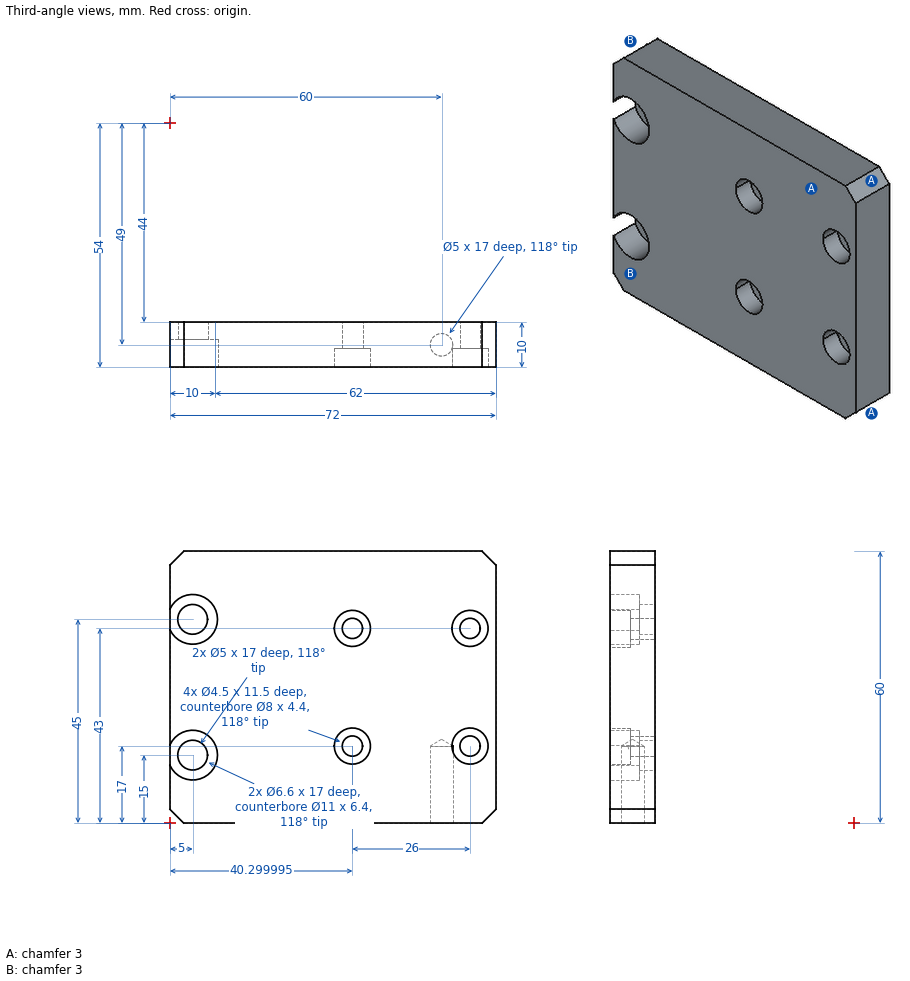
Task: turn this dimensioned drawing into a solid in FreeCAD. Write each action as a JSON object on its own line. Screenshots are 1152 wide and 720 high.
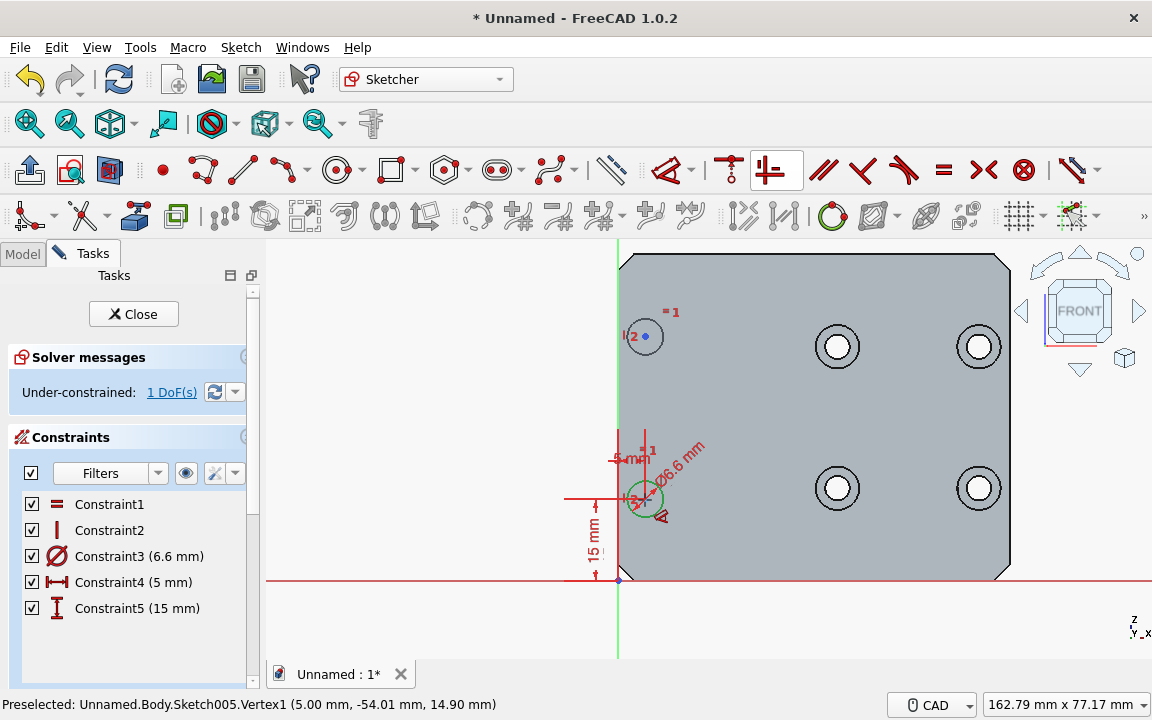
{"action": "left_click", "coordinate": [645, 337]}
{"action": "left_click", "coordinate": [584, 403]}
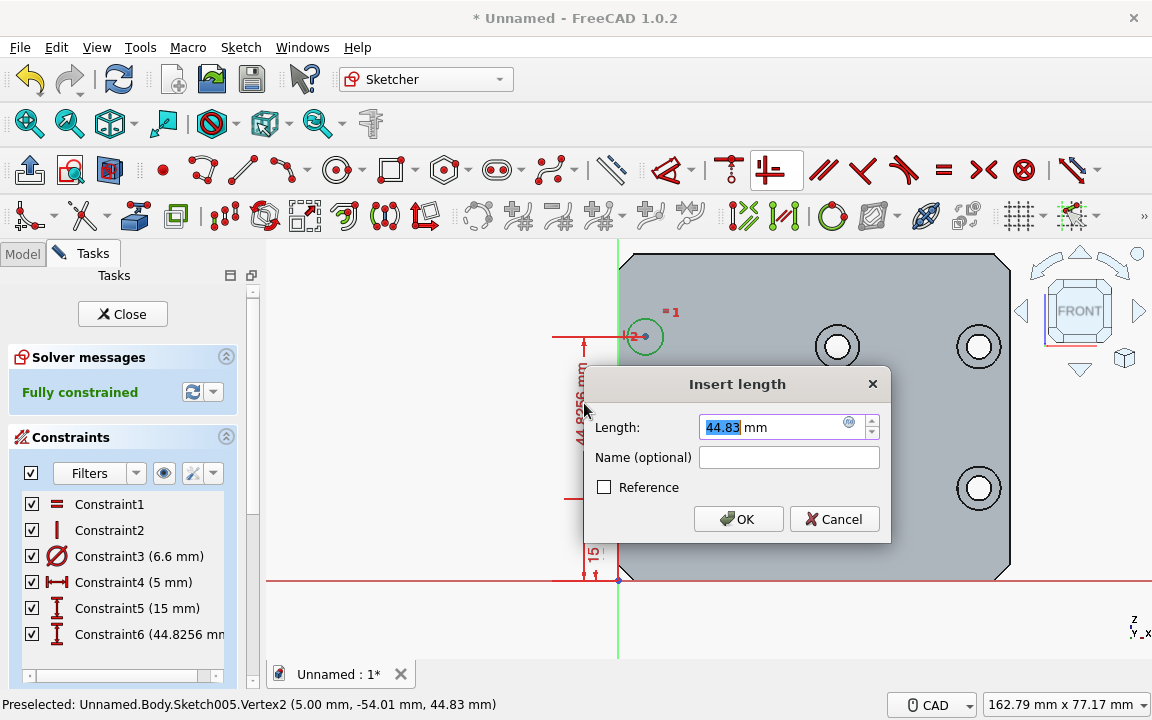
{"action": "type", "text": "45"}
{"action": "key", "text": "Return"}
{"action": "key", "text": "Escape"}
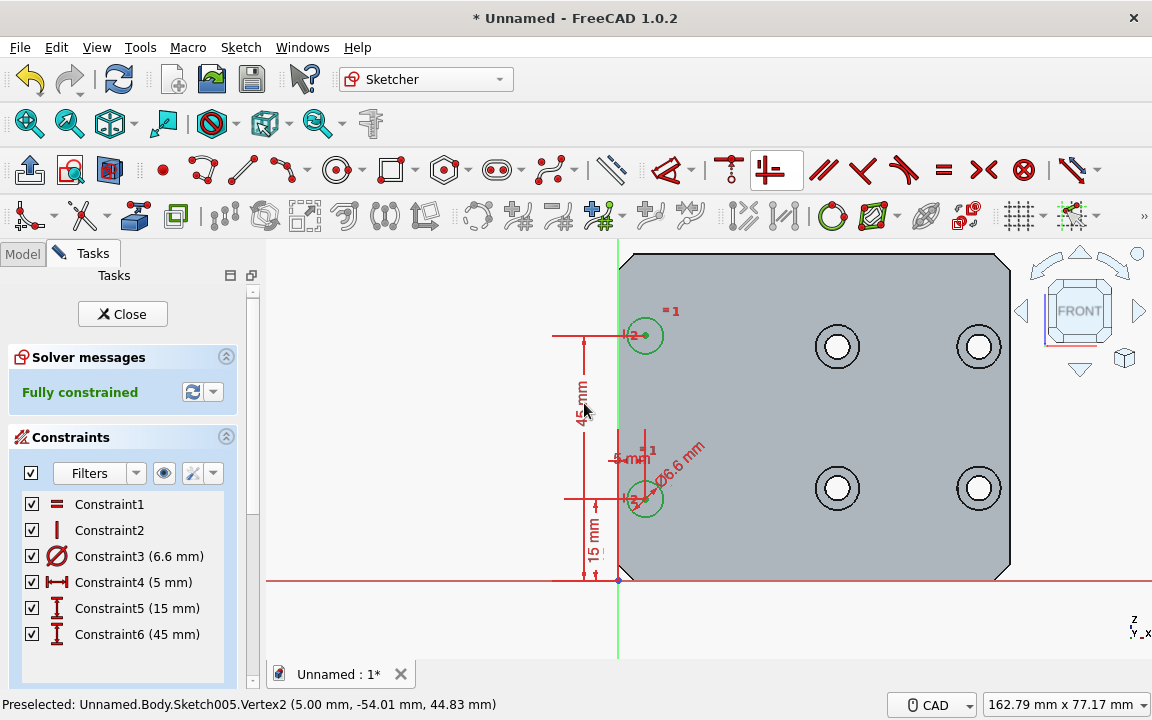
{"action": "left_click", "coordinate": [123, 314]}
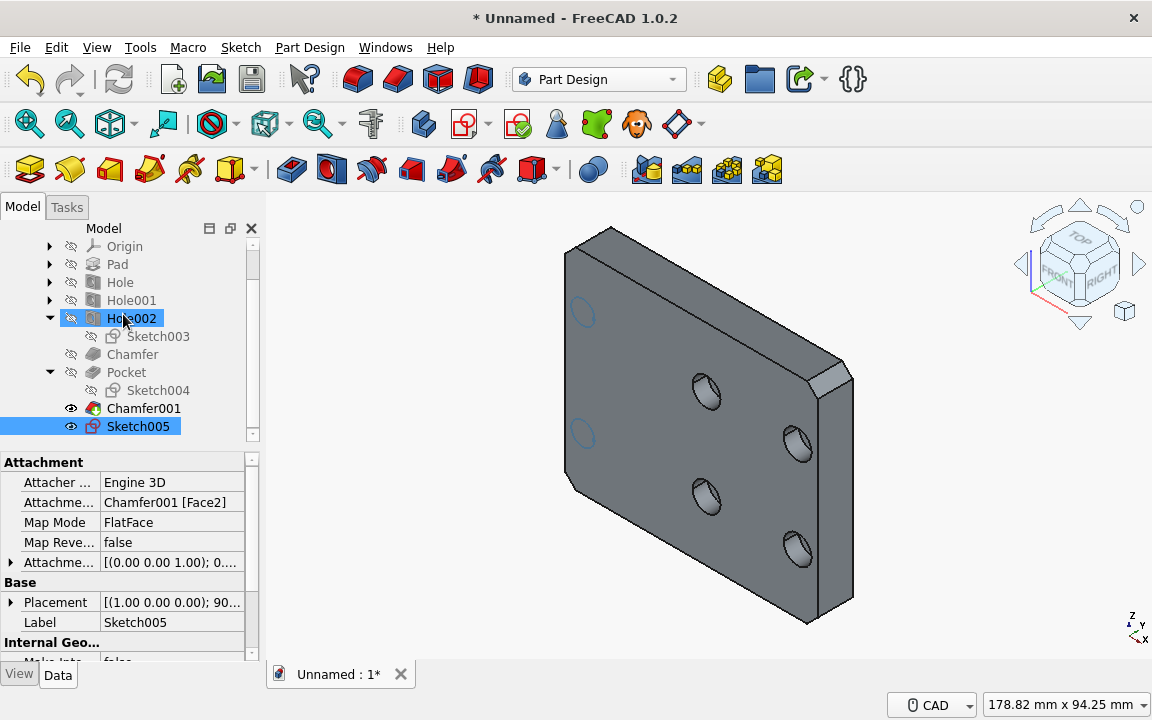
{"action": "left_click", "coordinate": [332, 170]}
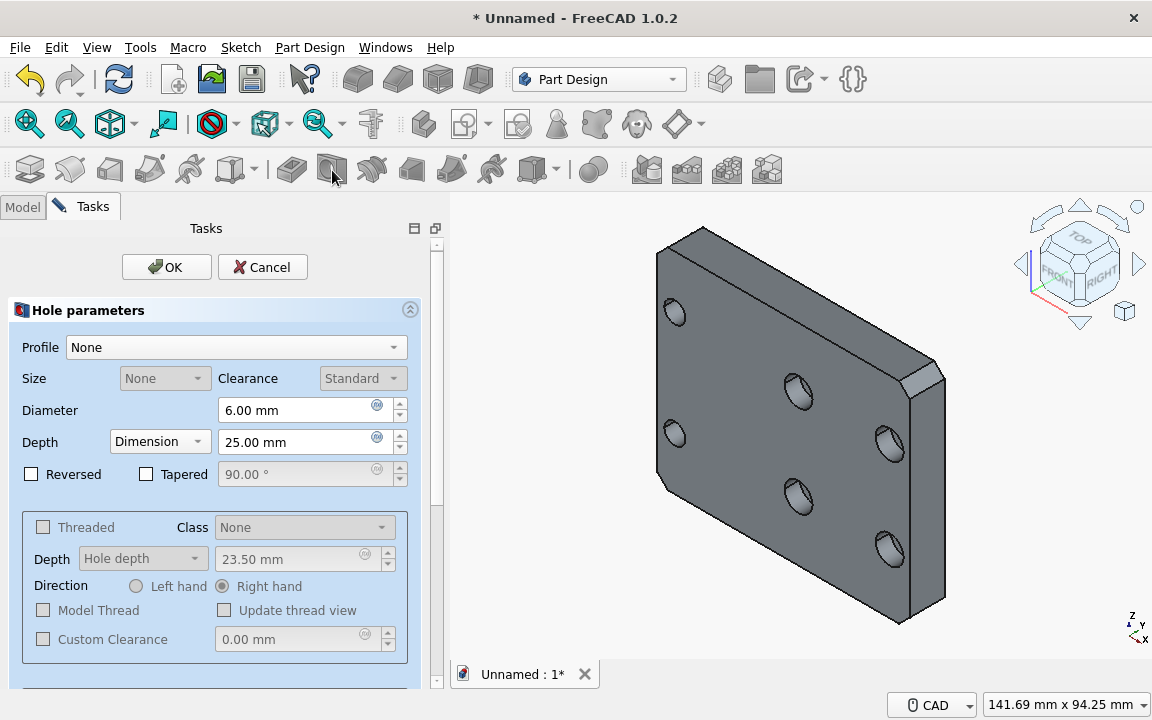
{"action": "triple_click", "coordinate": [305, 410]}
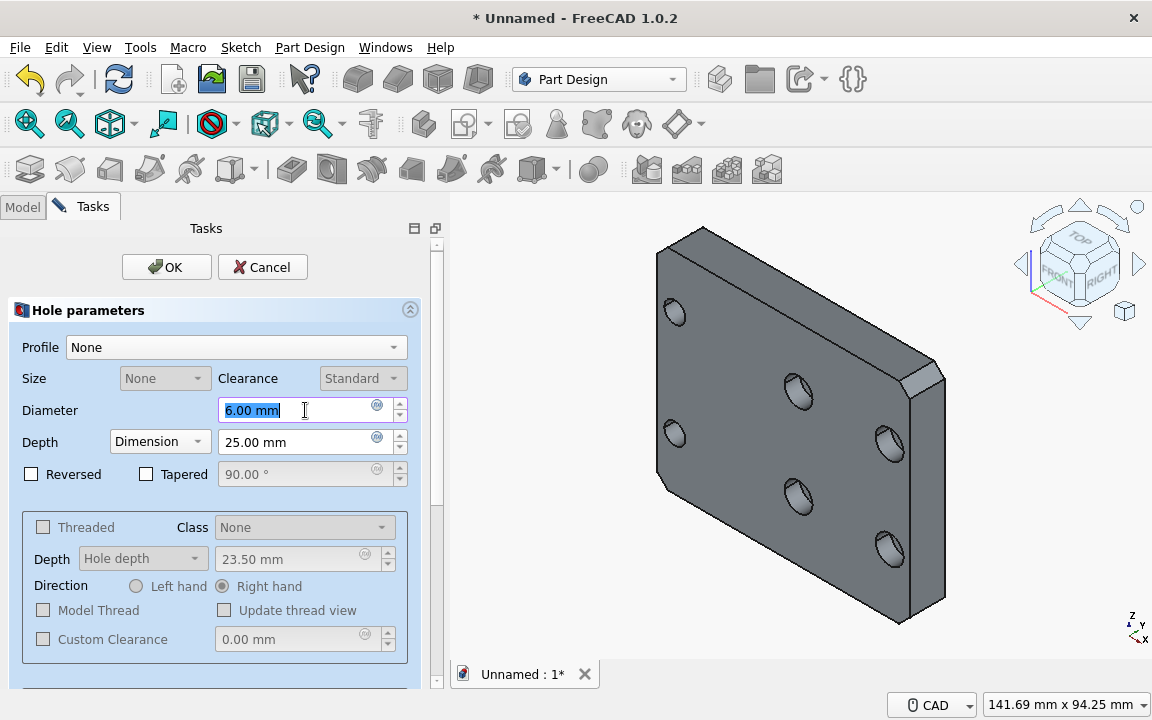
{"action": "type", "text": "6.6"}
{"action": "key", "text": "Tab"}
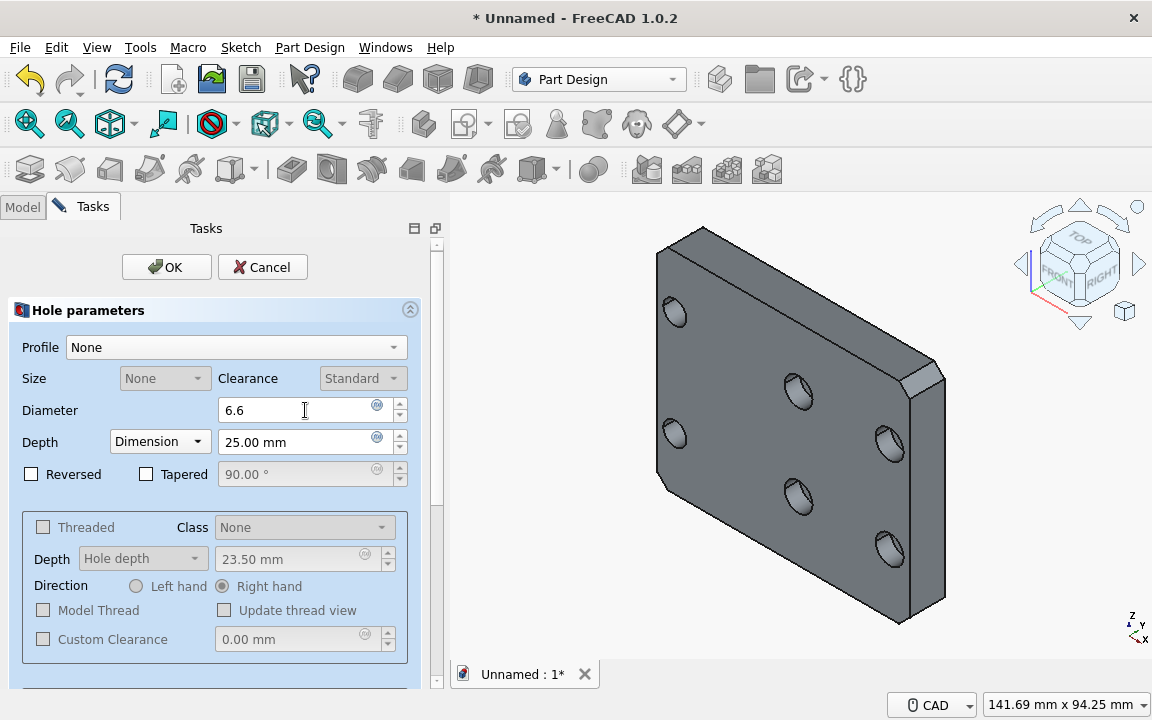
{"action": "triple_click", "coordinate": [305, 442]}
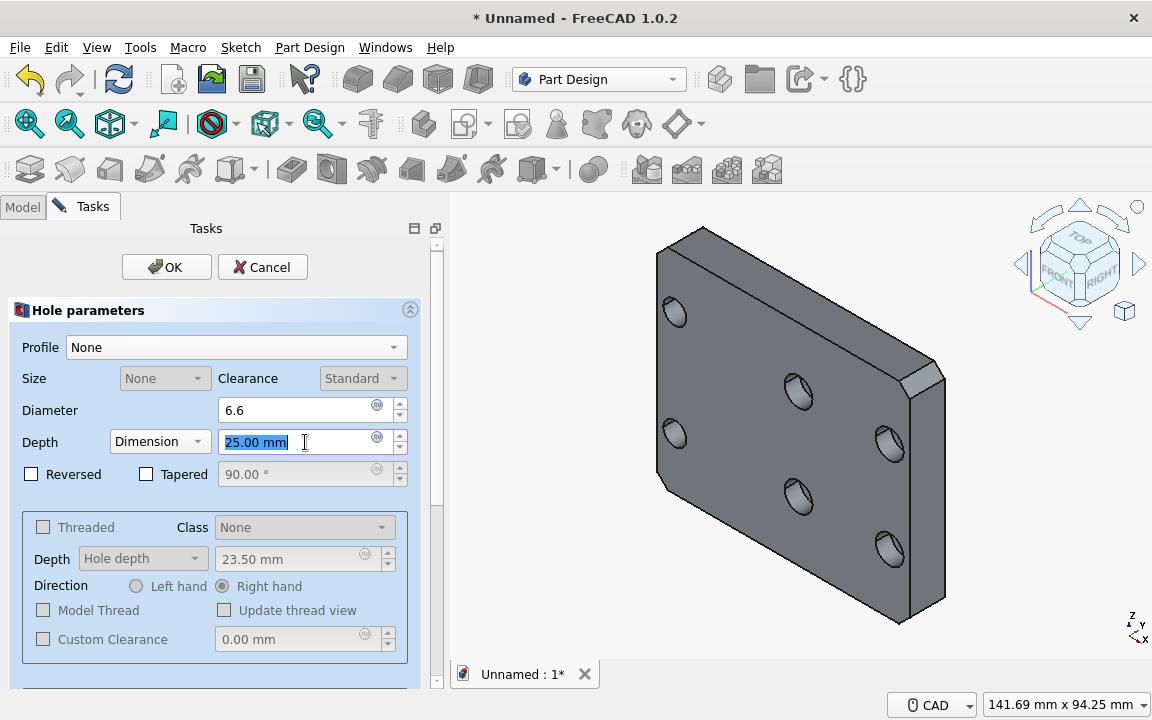
{"action": "type", "text": "17"}
{"action": "key", "text": "Tab"}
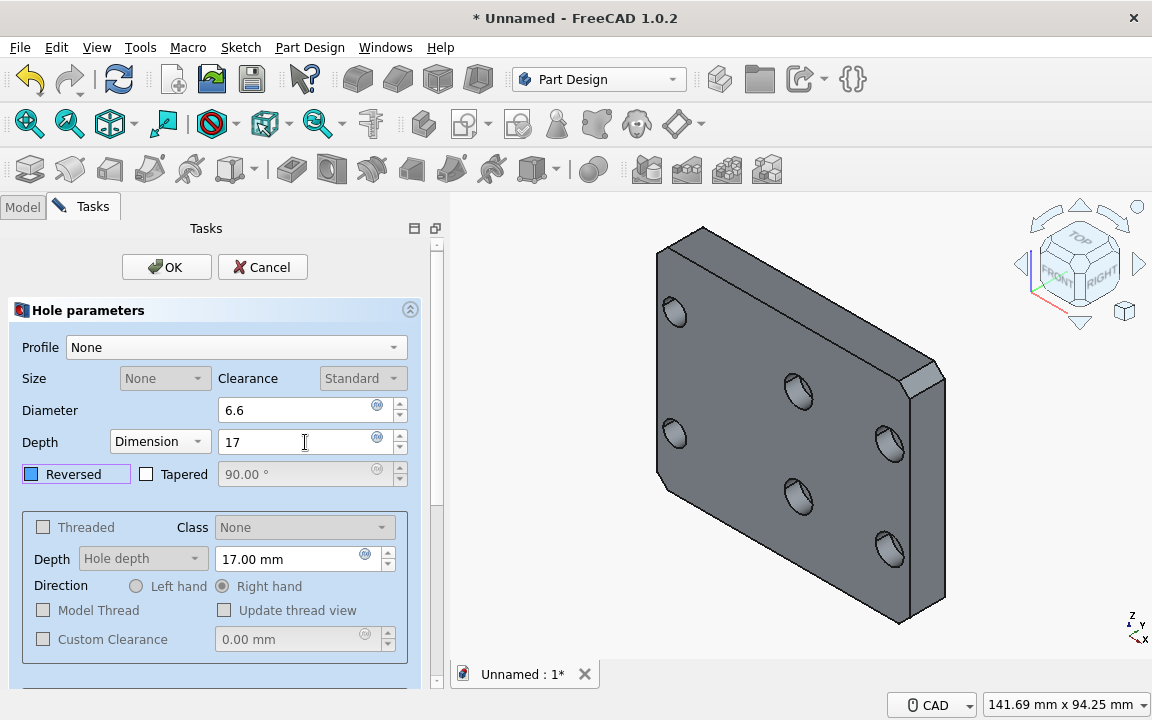
{"action": "scroll", "coordinate": [437, 463], "scroll_direction": "down", "scroll_amount": 2}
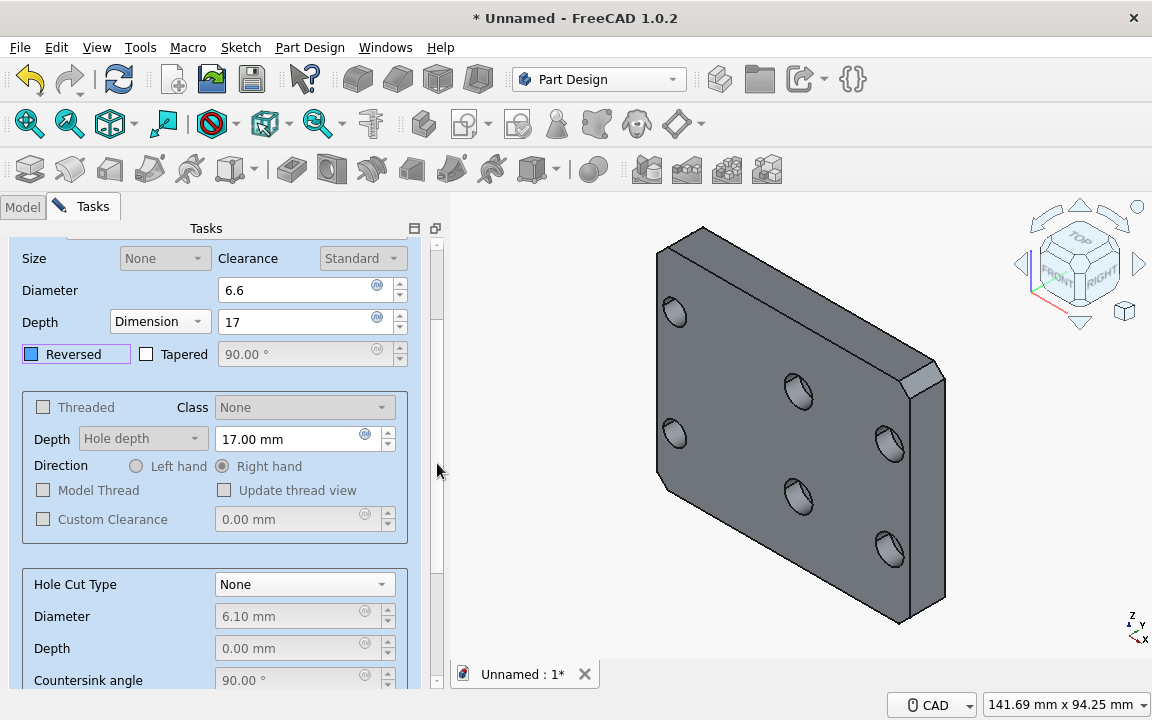
{"action": "left_click", "coordinate": [306, 584]}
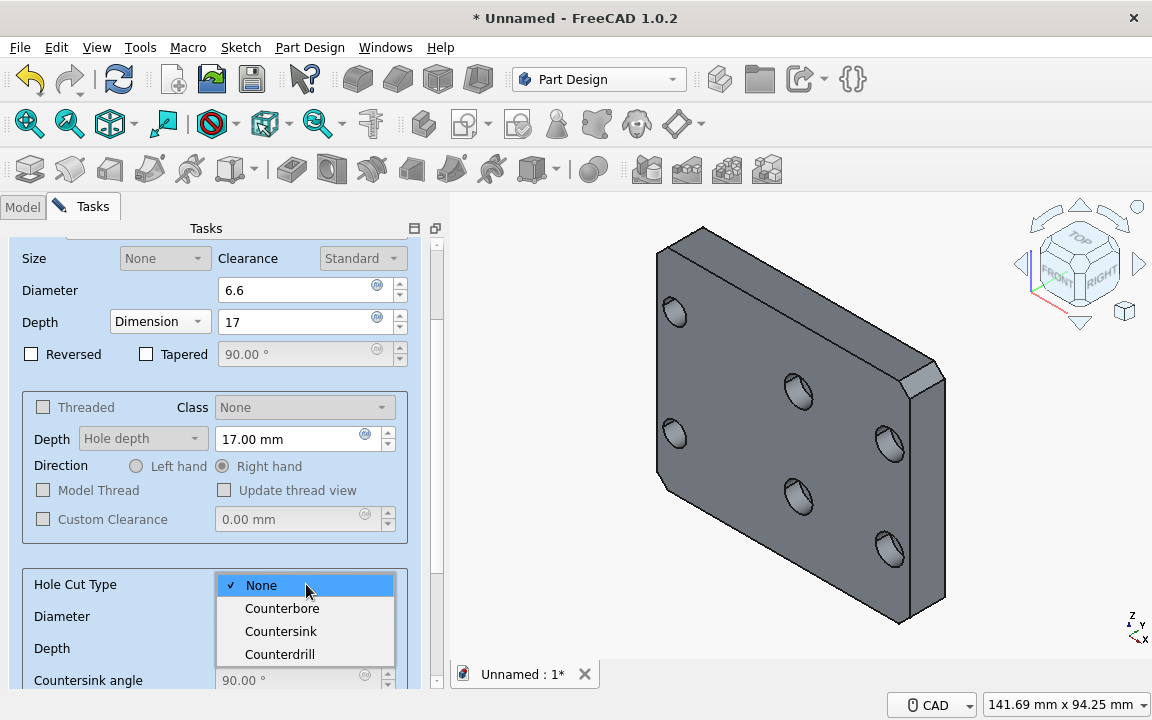
{"action": "left_click", "coordinate": [304, 608]}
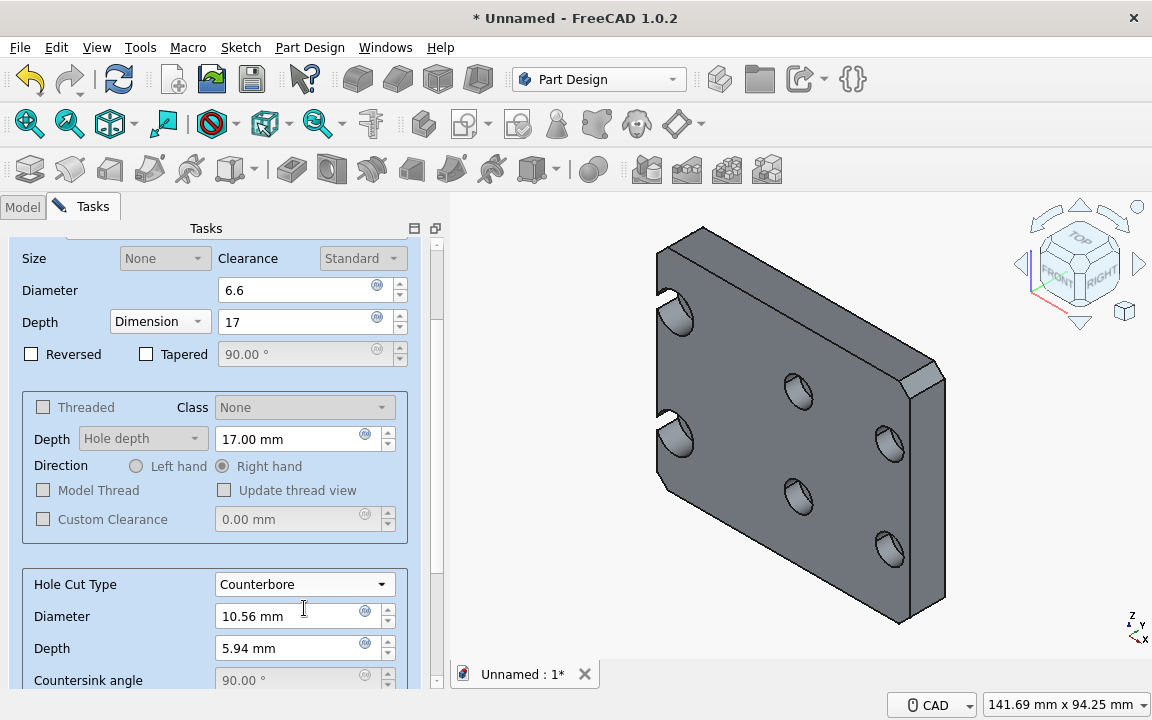
{"action": "triple_click", "coordinate": [298, 616]}